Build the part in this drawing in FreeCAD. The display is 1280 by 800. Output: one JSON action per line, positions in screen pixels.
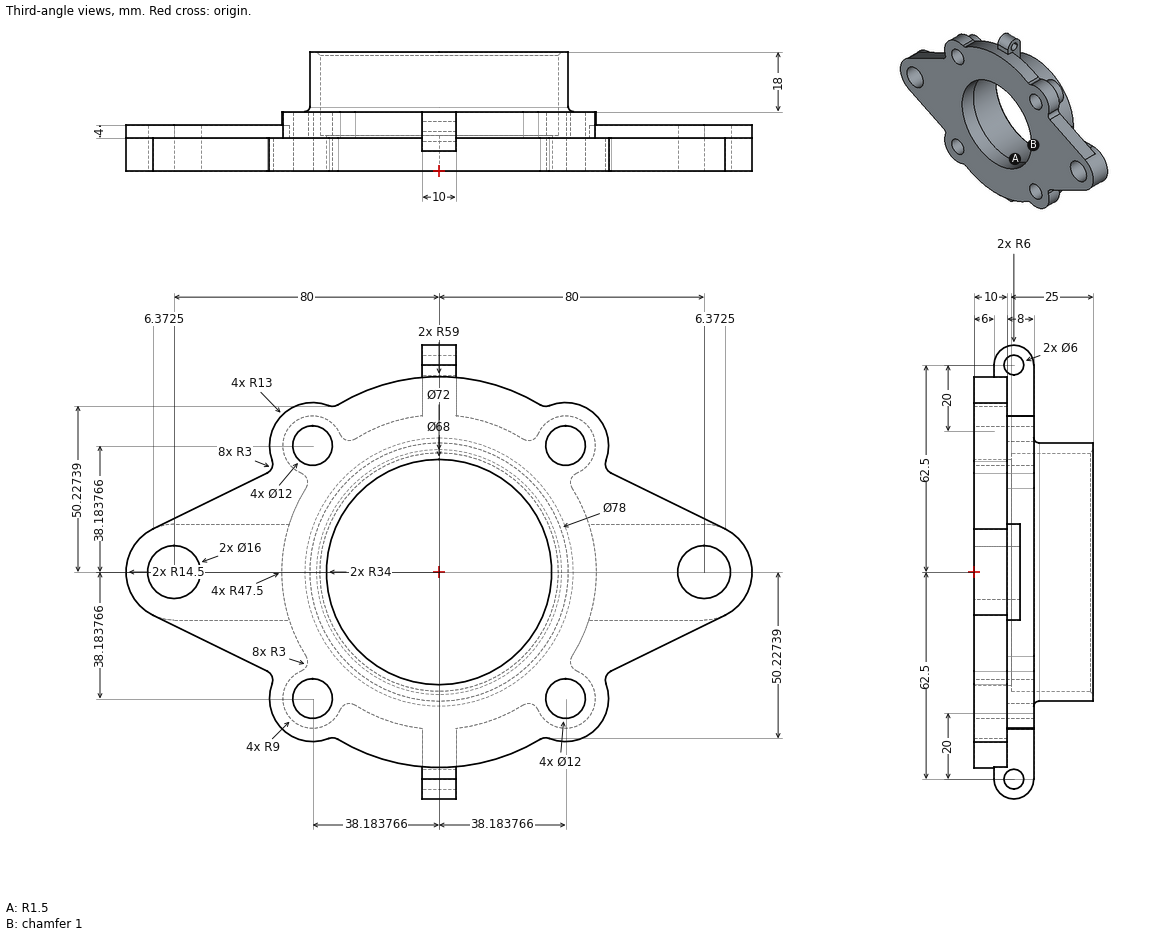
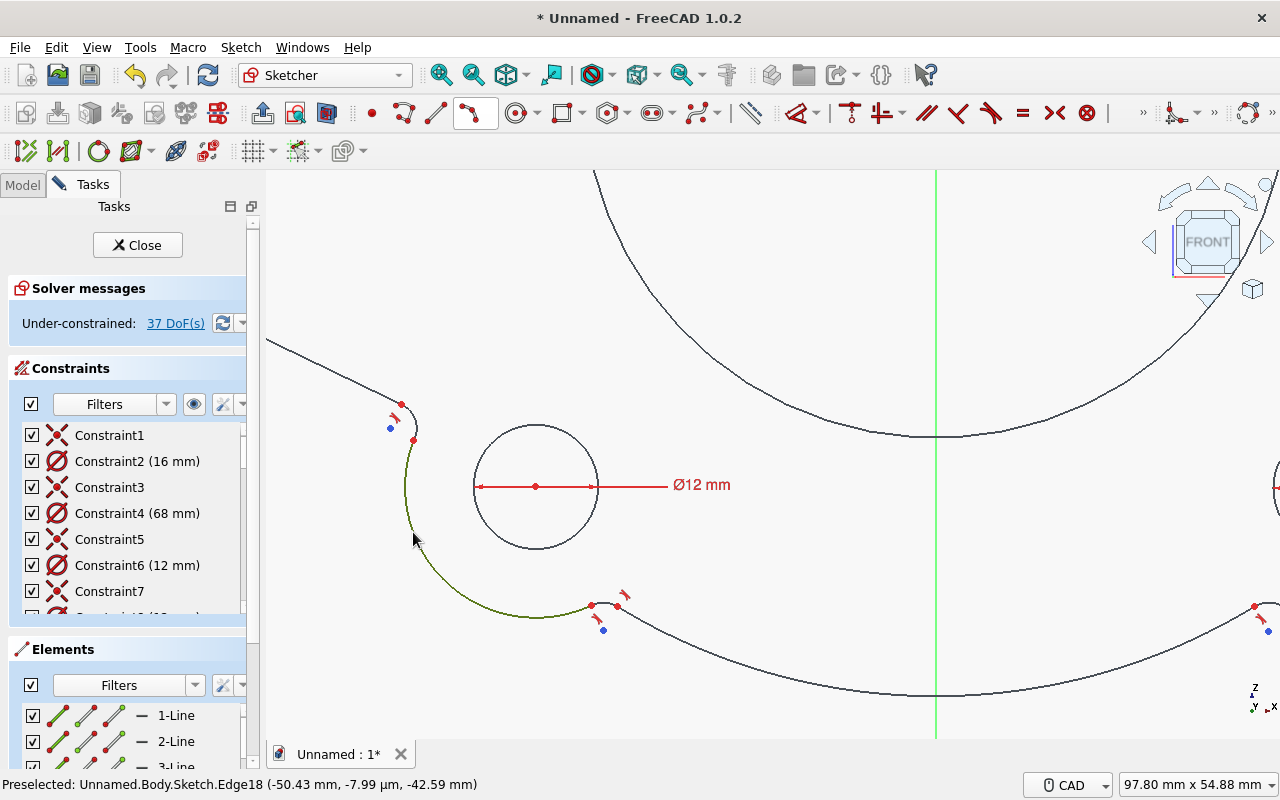
{"action": "left_click", "coordinate": [417, 429]}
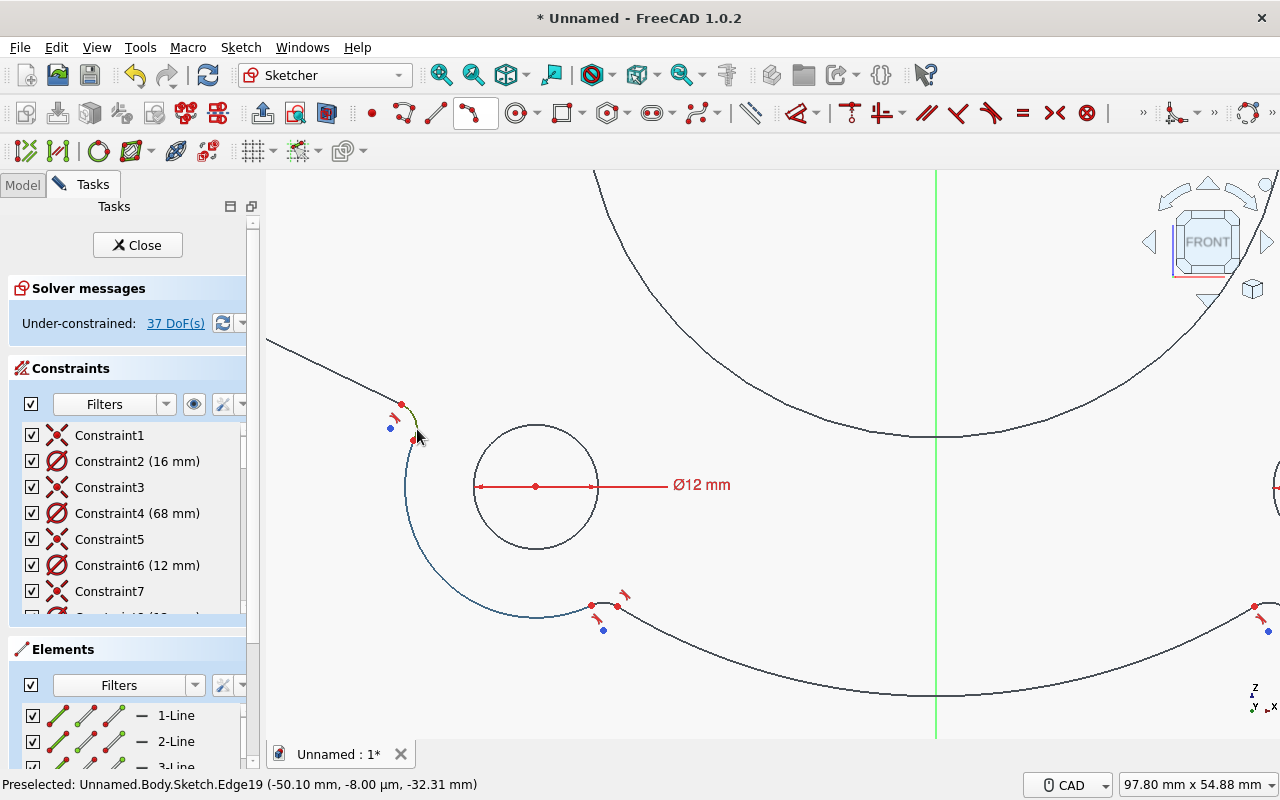
{"action": "left_click", "coordinate": [992, 114]}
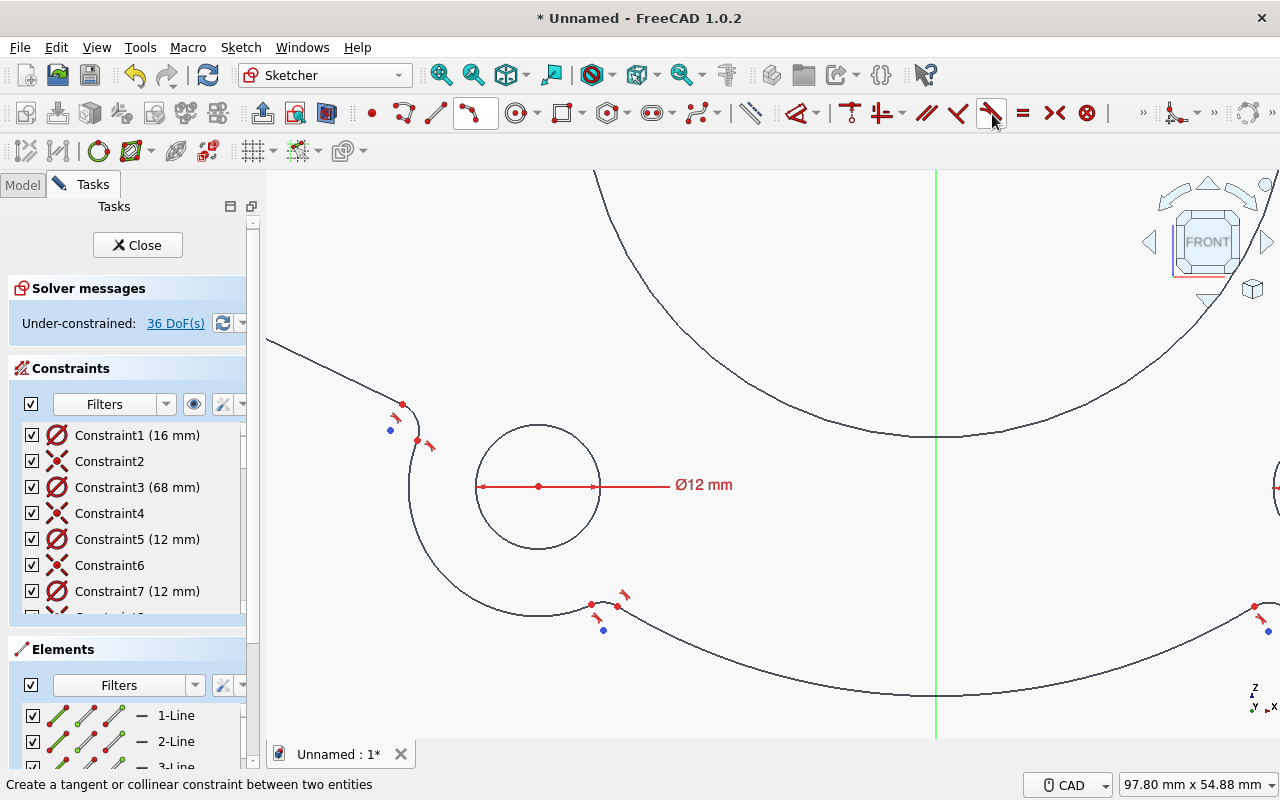
{"action": "left_click", "coordinate": [688, 335]}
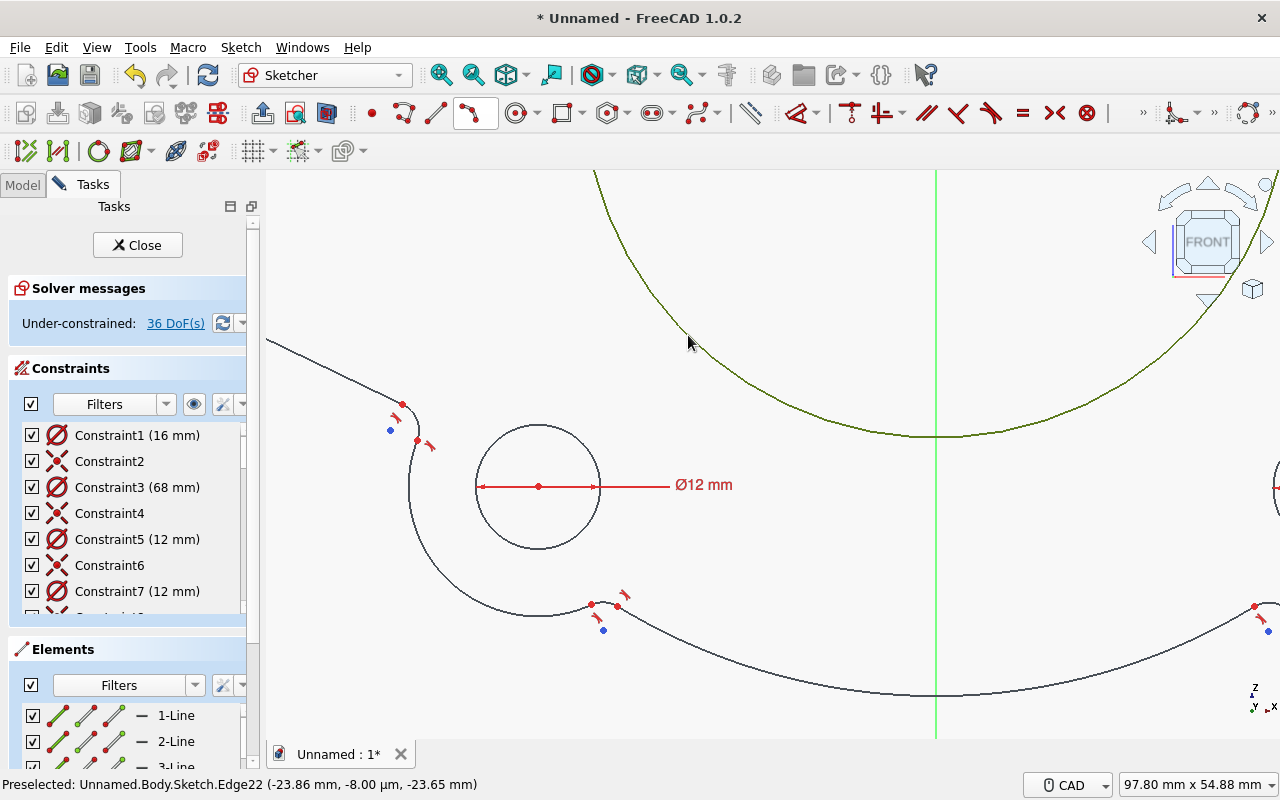
{"action": "scroll", "coordinate": [605, 612], "scroll_direction": "down", "scroll_amount": 6}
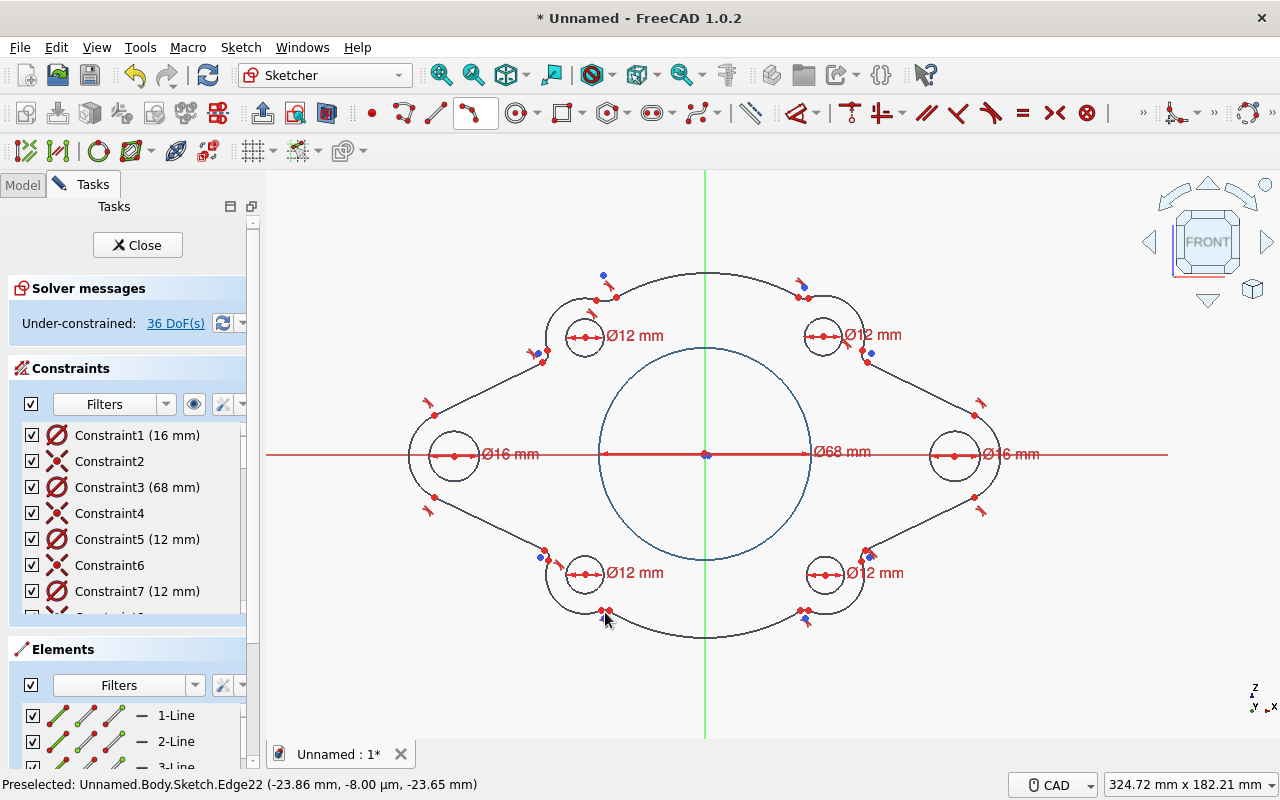
{"action": "left_click", "coordinate": [746, 277]}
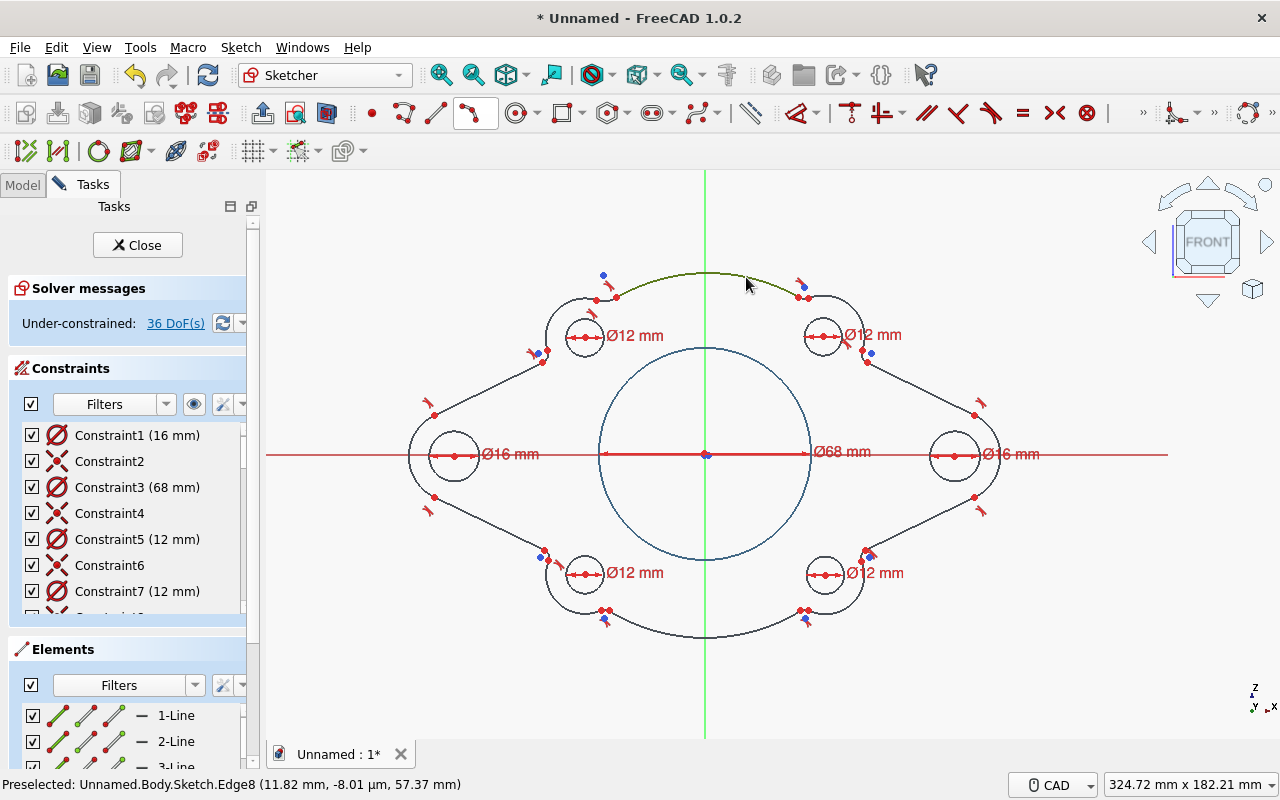
{"action": "left_click", "coordinate": [850, 114]}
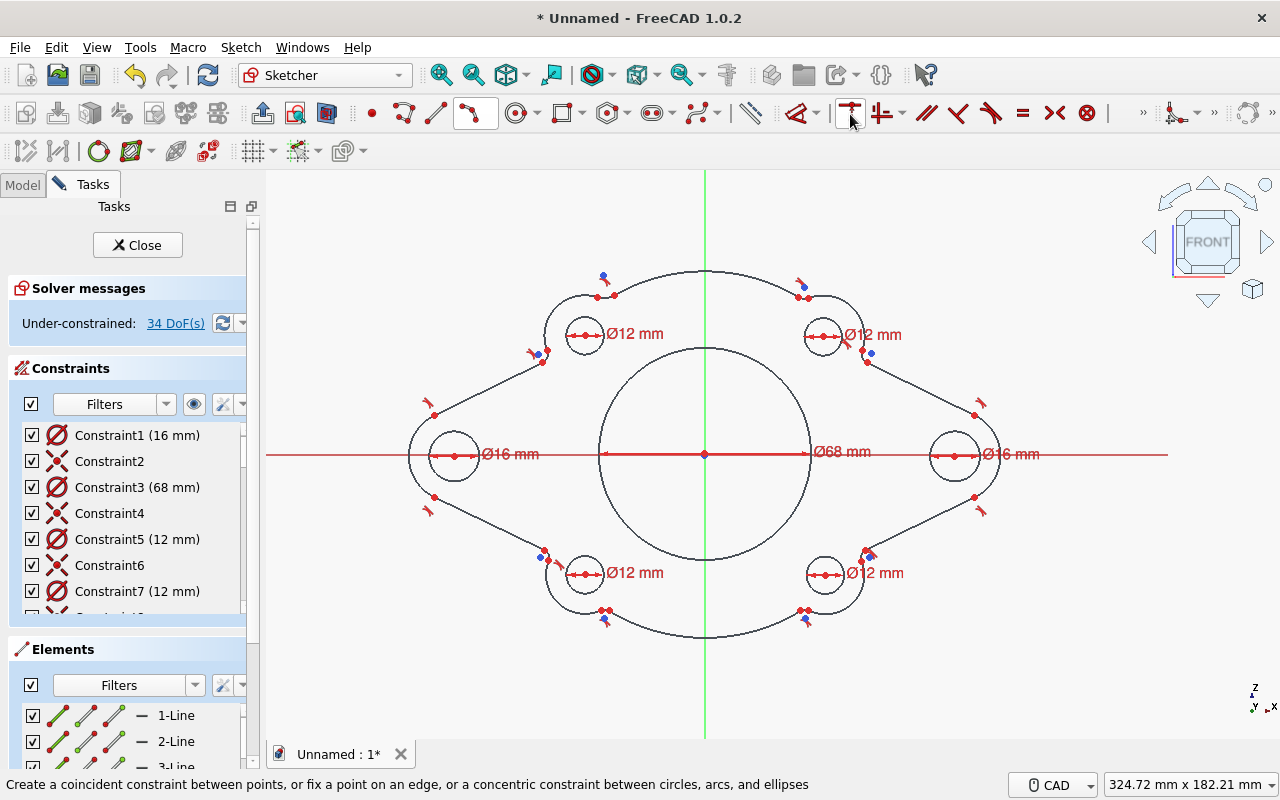
{"action": "scroll", "coordinate": [705, 455], "scroll_direction": "up", "scroll_amount": 8}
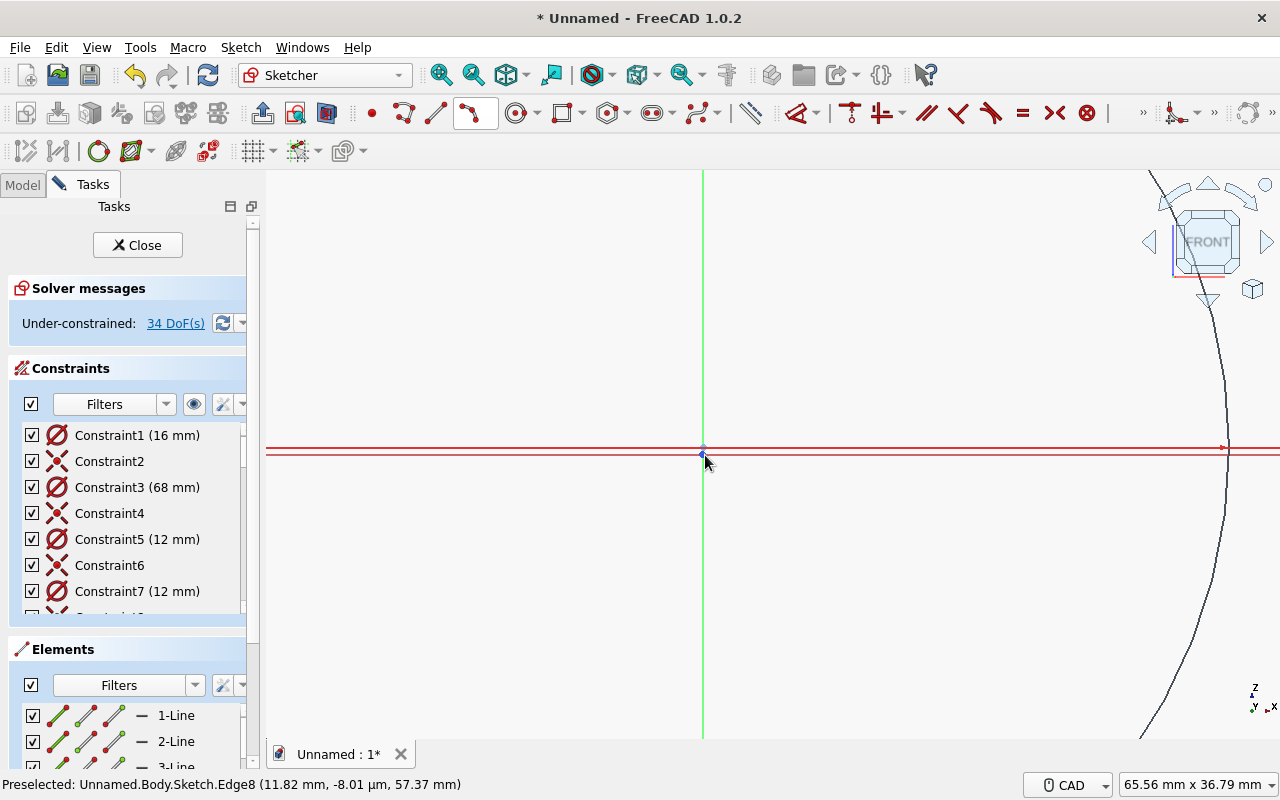
{"action": "left_click_drag", "start_coordinate": [693, 438], "coordinate": [713, 465]}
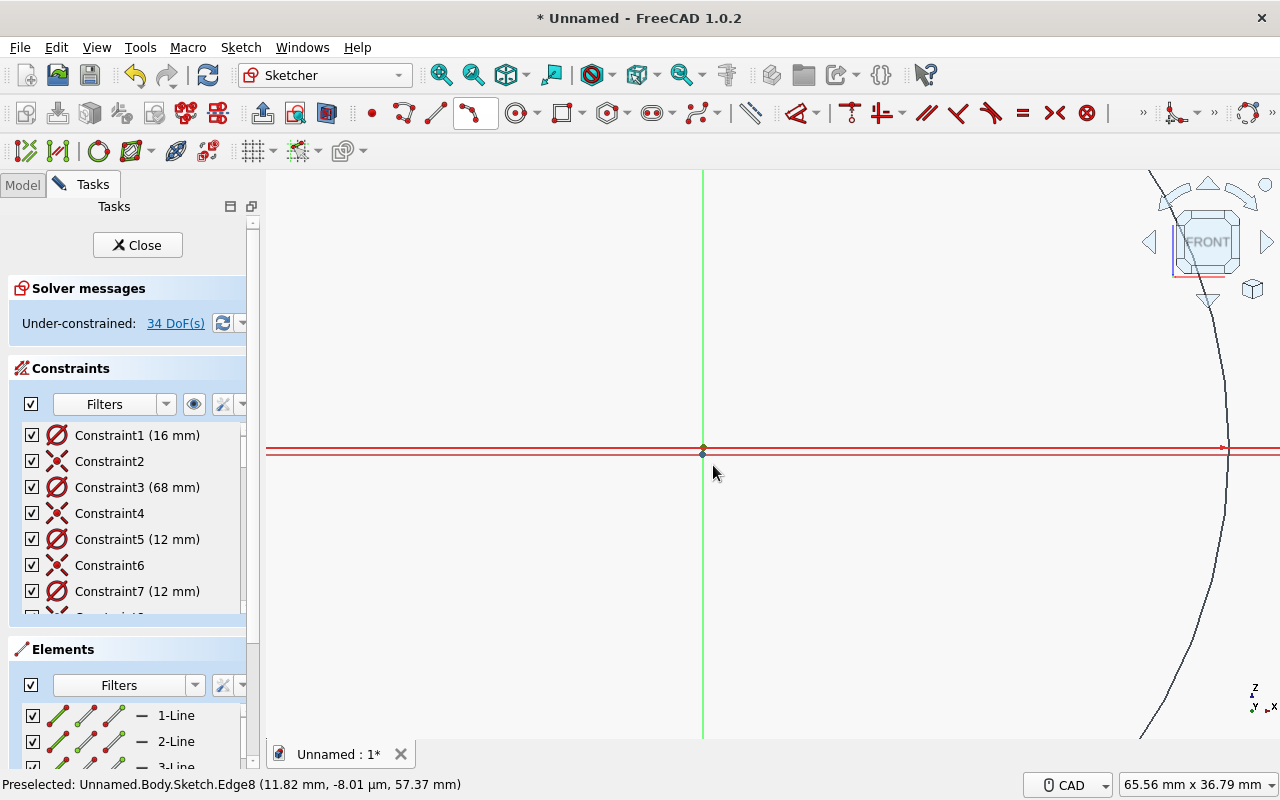
{"action": "left_click", "coordinate": [850, 114]}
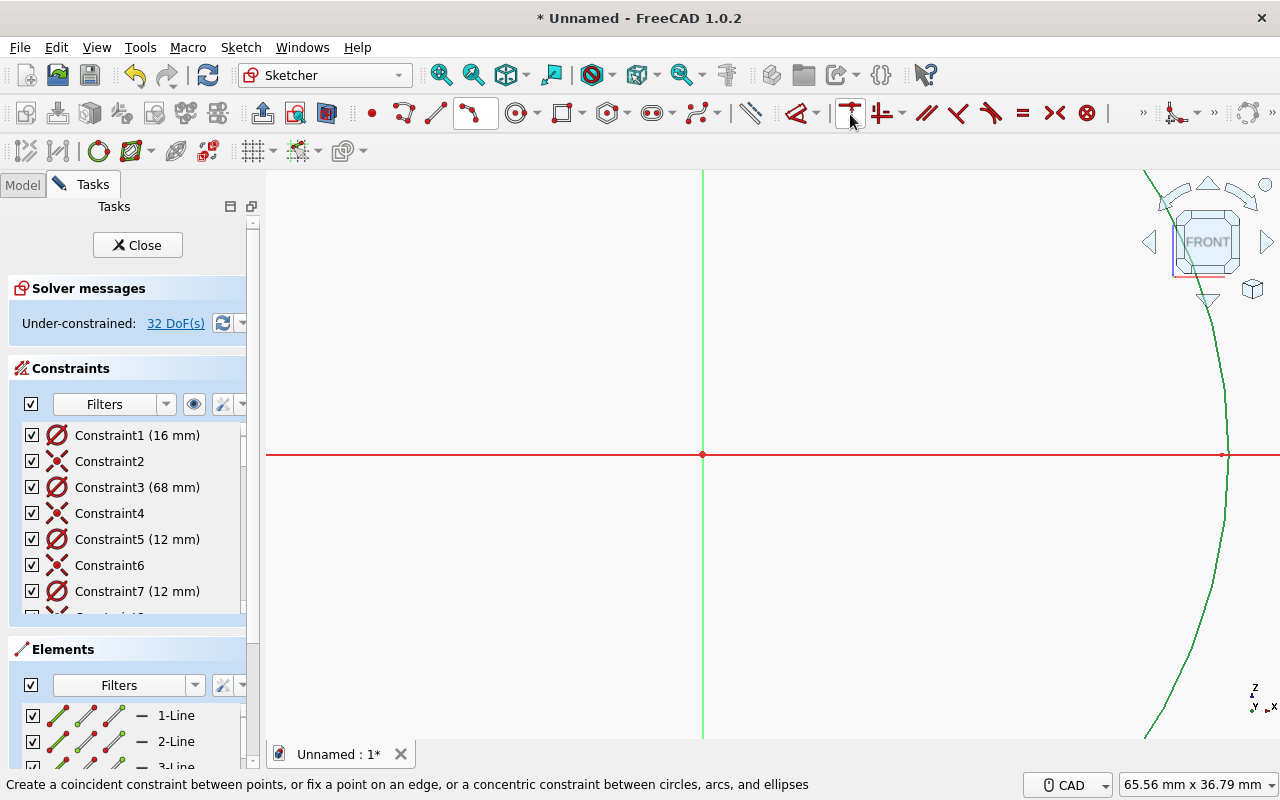
{"action": "scroll", "coordinate": [705, 454], "scroll_direction": "down", "scroll_amount": 8}